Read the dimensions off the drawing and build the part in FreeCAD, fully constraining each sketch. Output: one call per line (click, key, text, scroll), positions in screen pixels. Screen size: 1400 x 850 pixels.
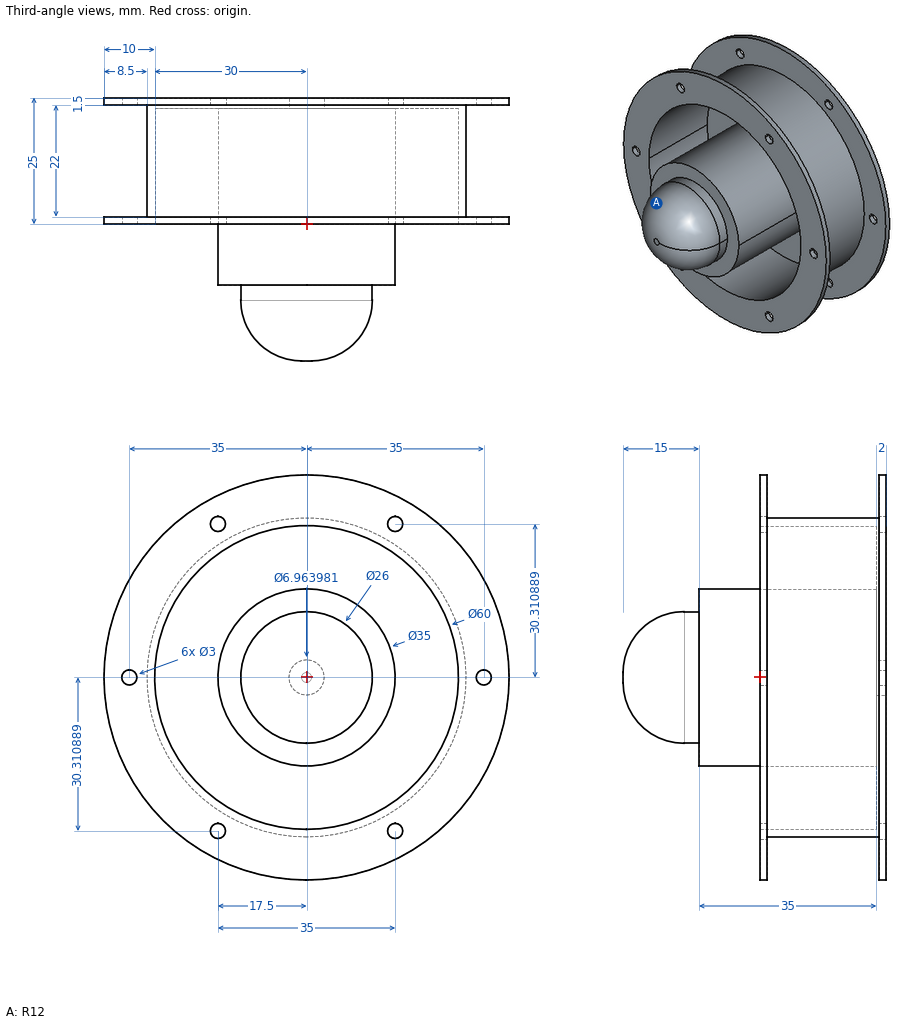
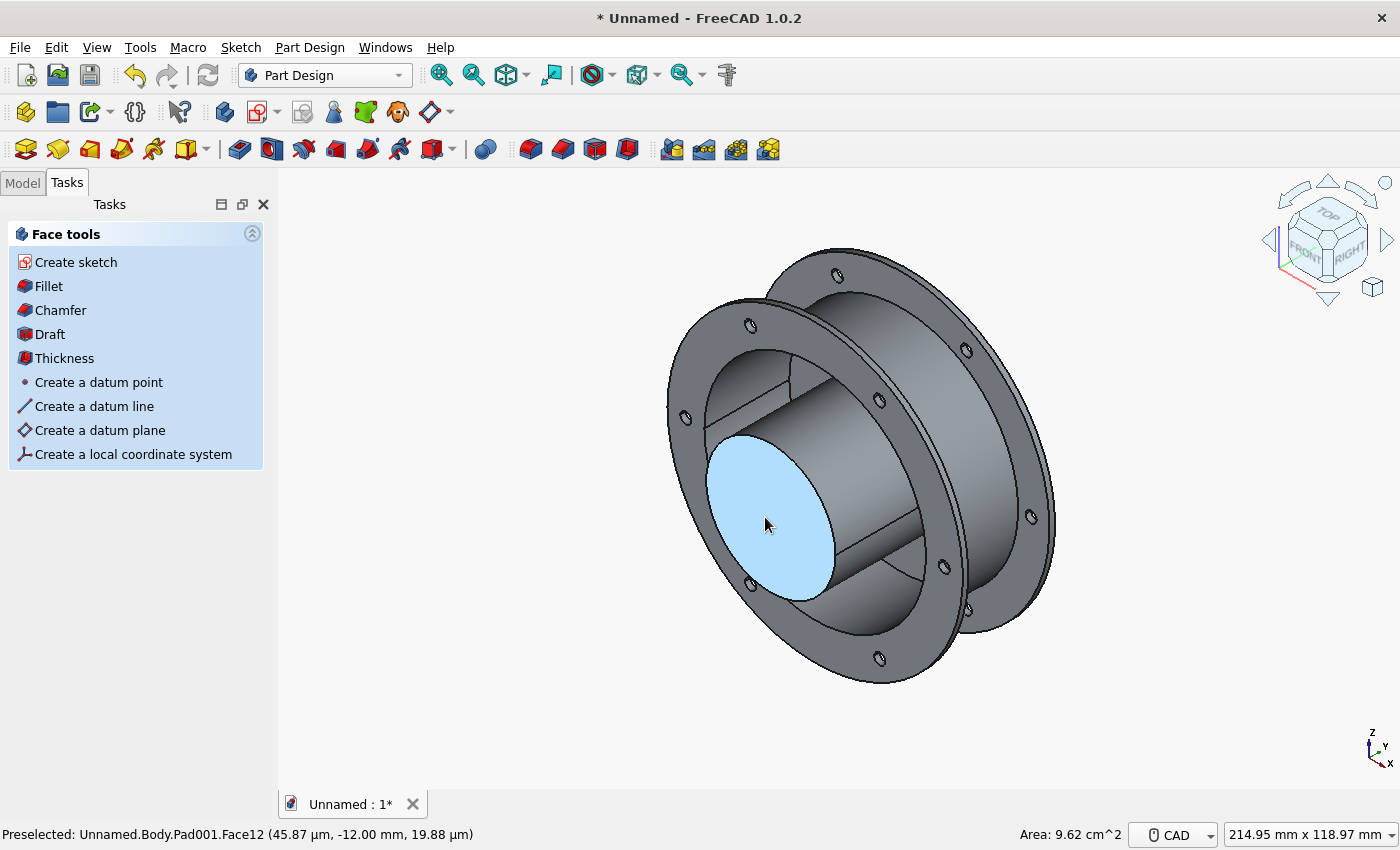
click(258, 112)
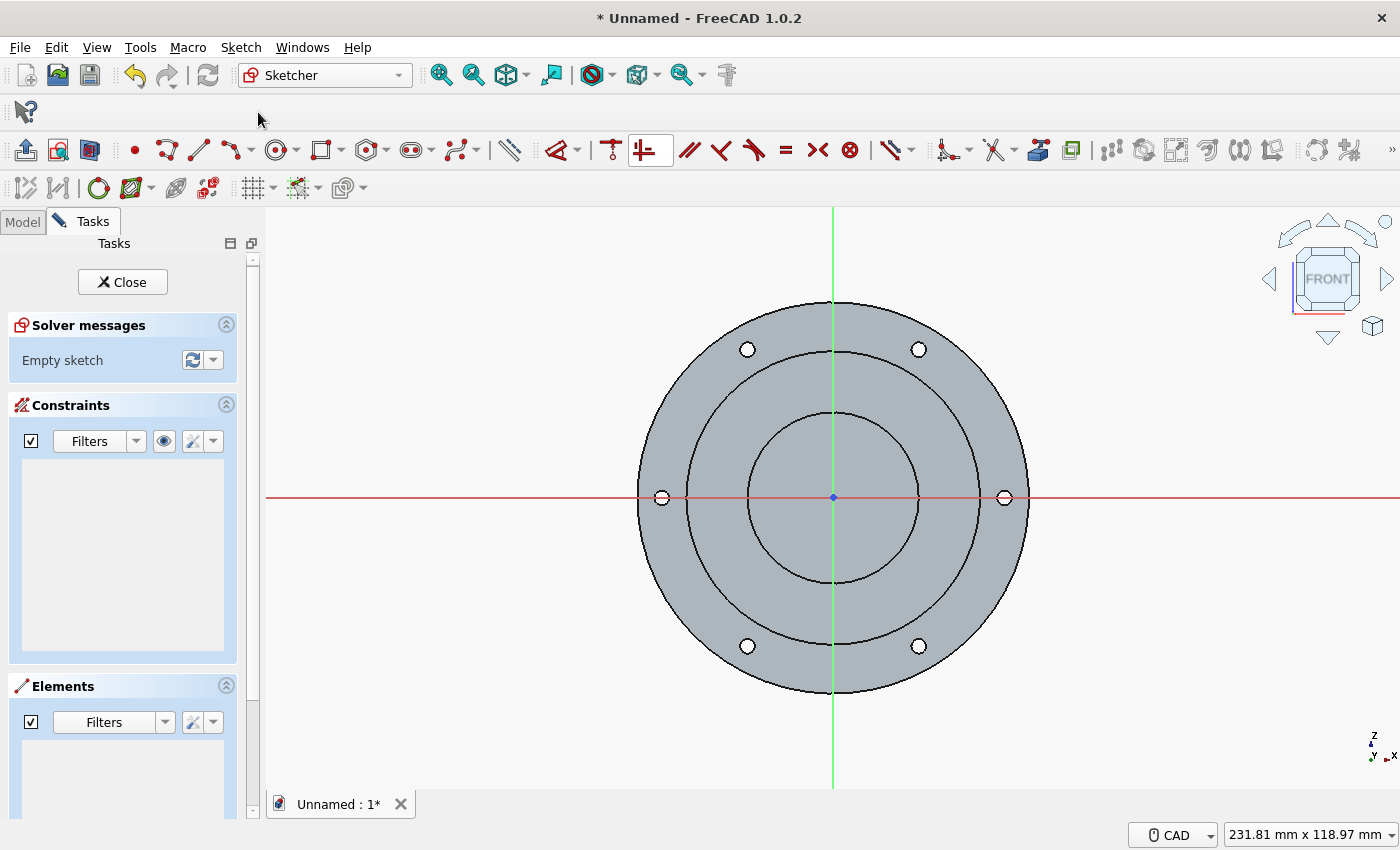
scroll(873, 498, up, 5)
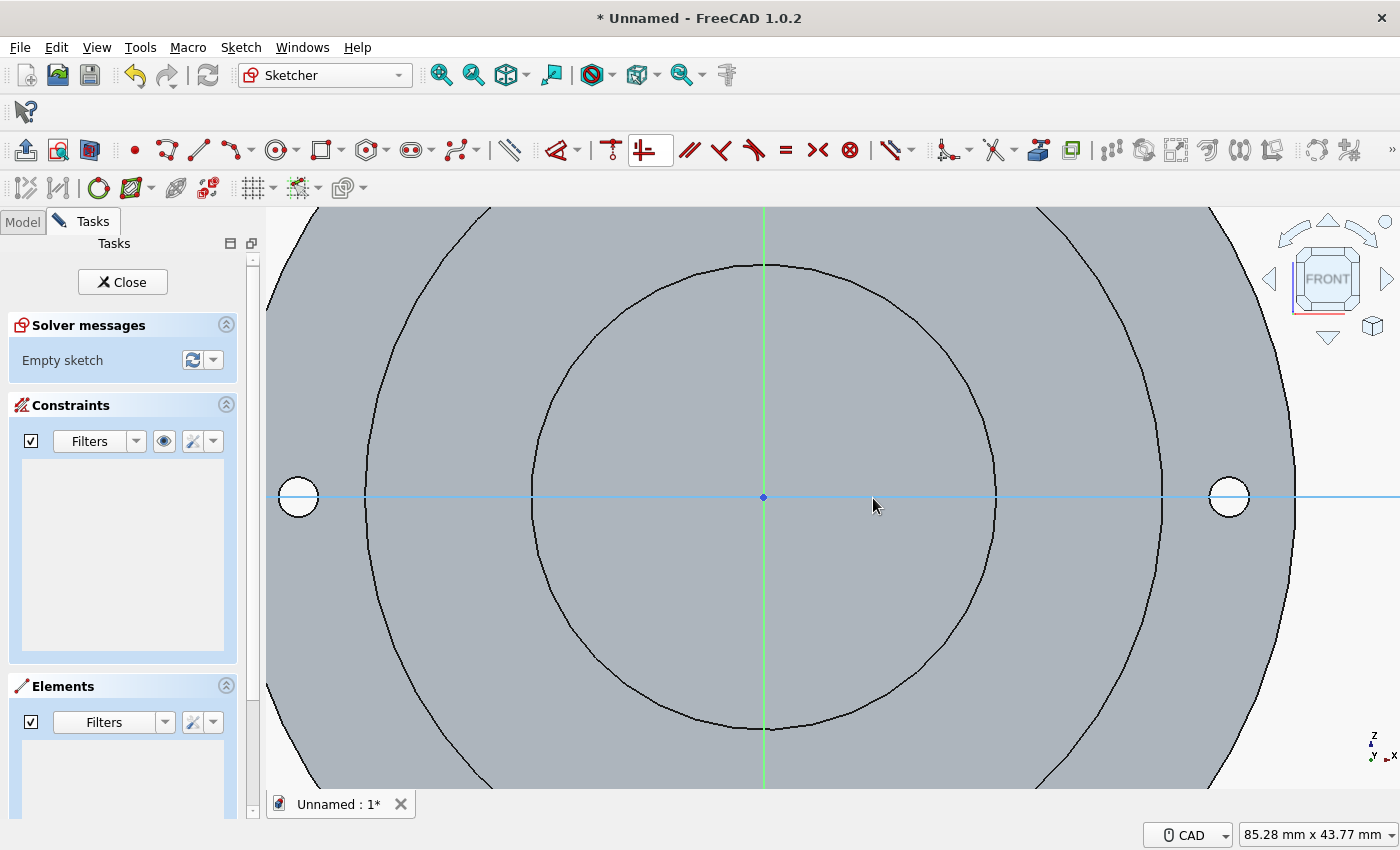
click(276, 150)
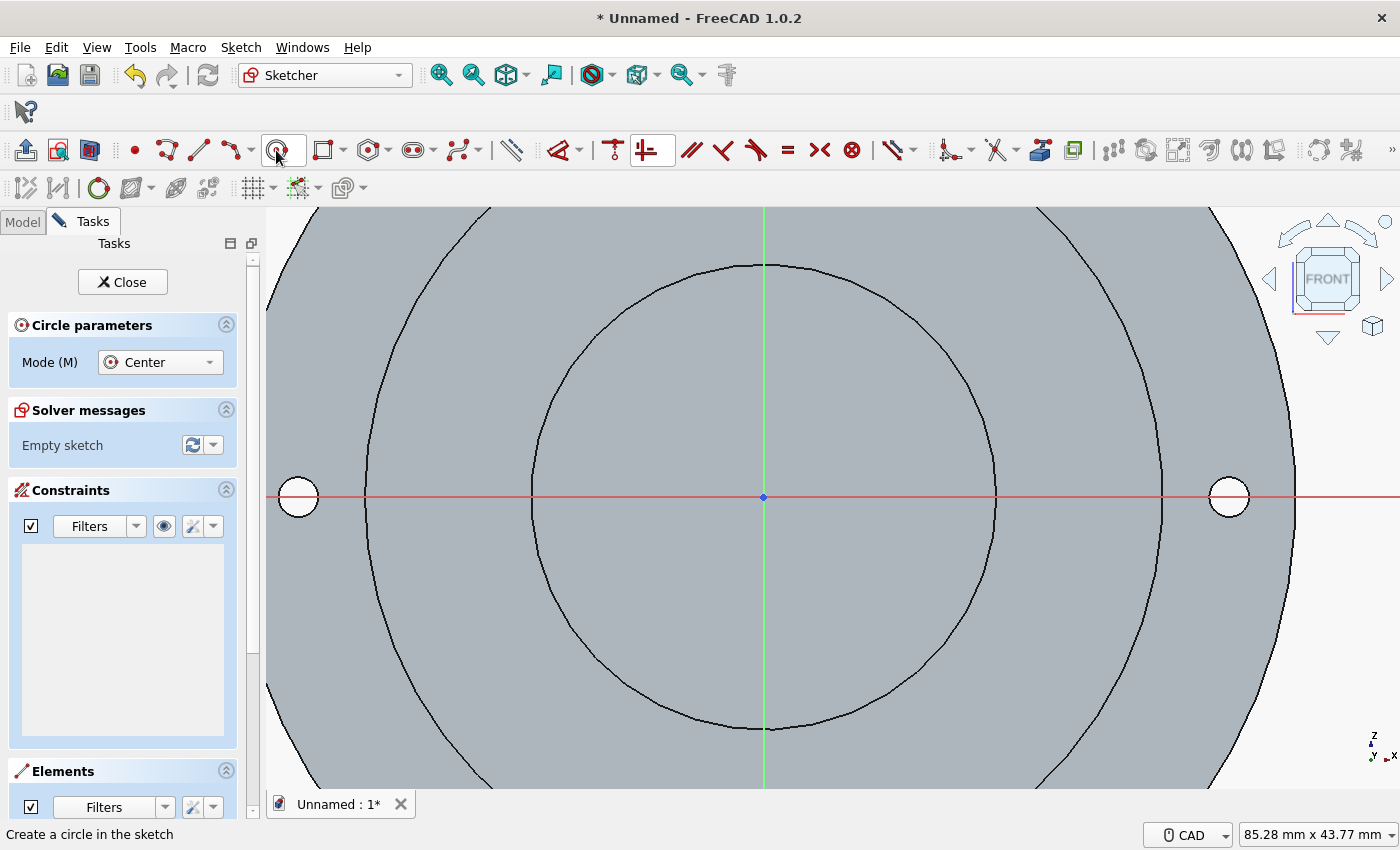
click(764, 497)
click(886, 375)
key(Escape)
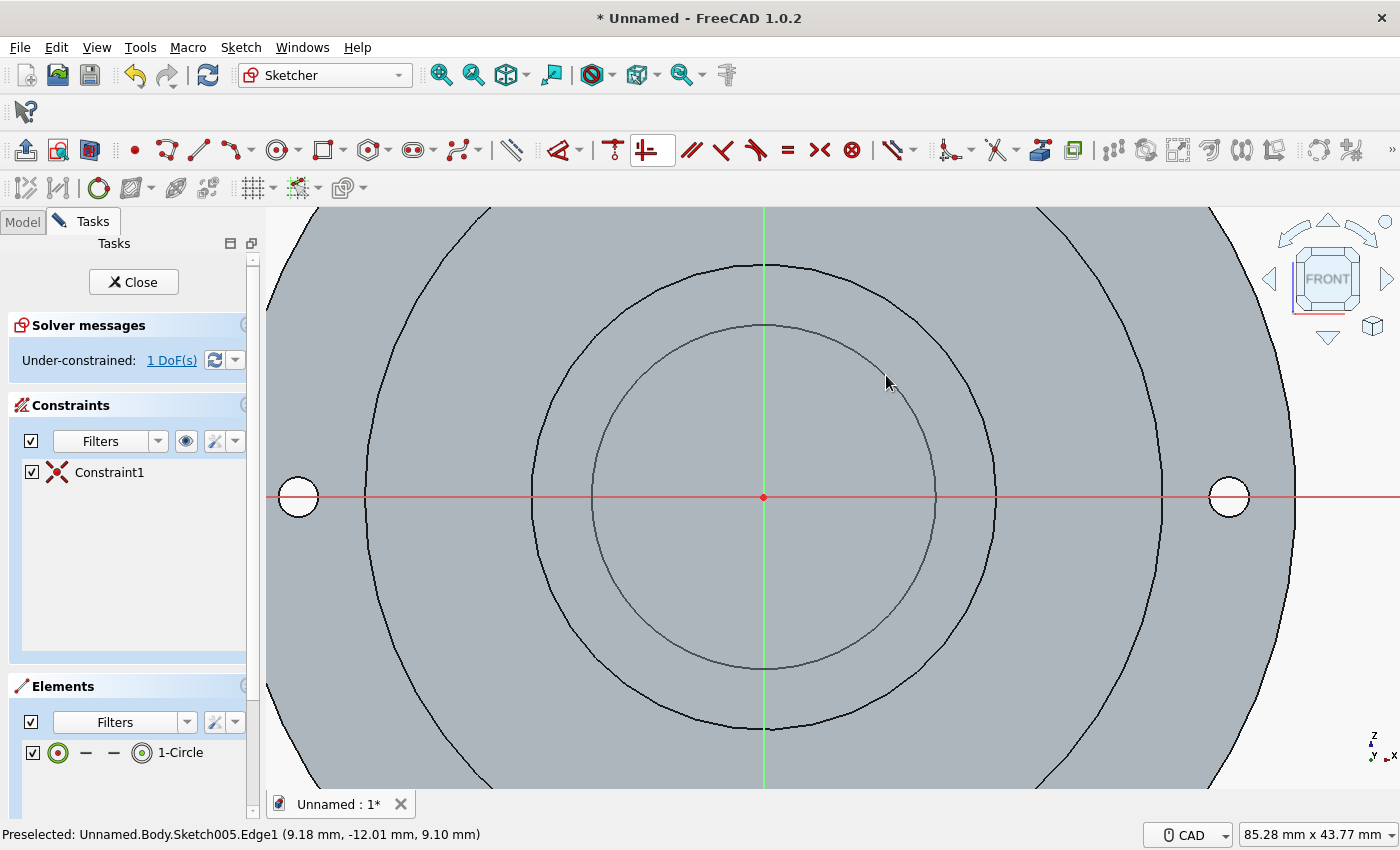
click(558, 150)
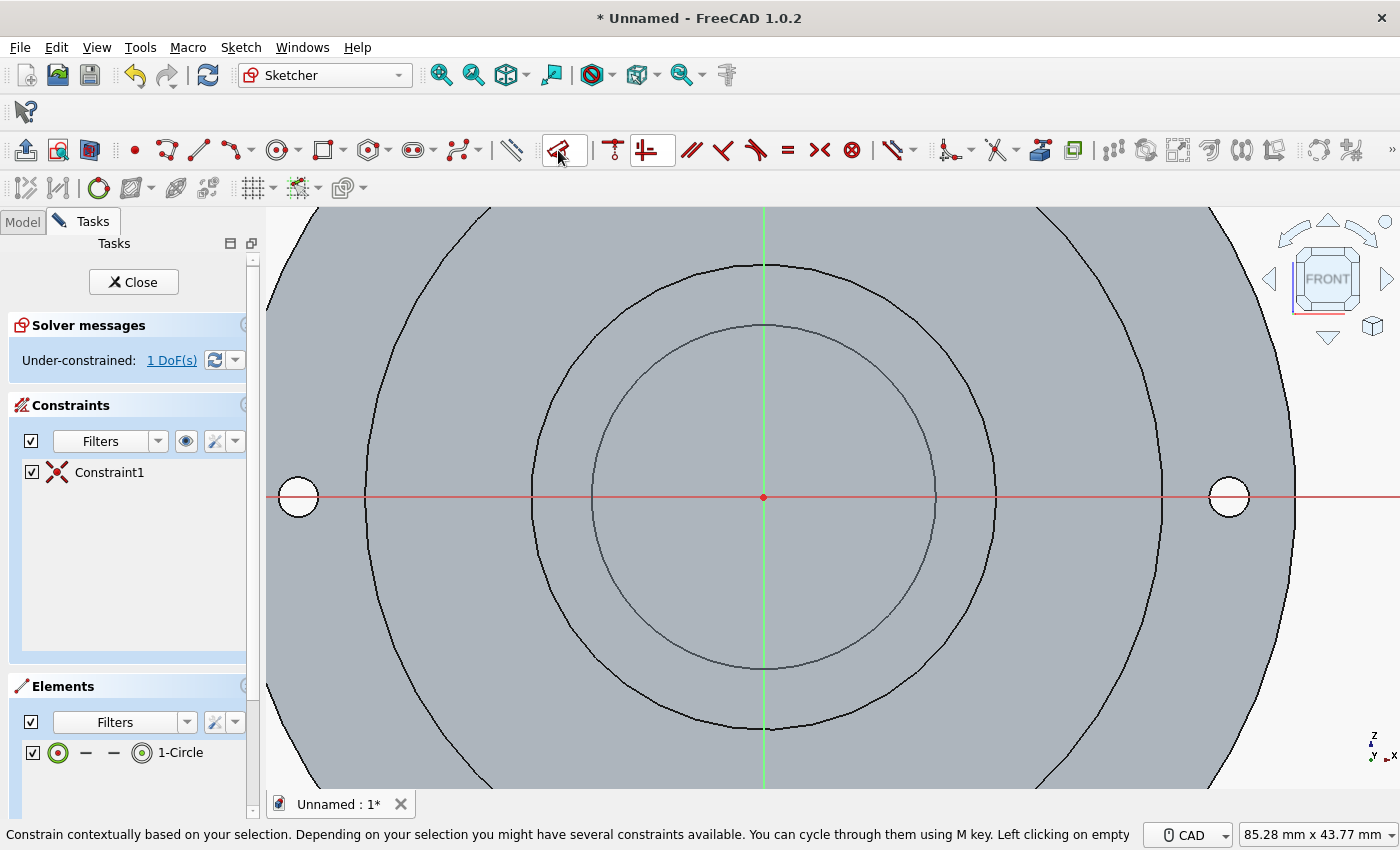
click(885, 375)
click(908, 352)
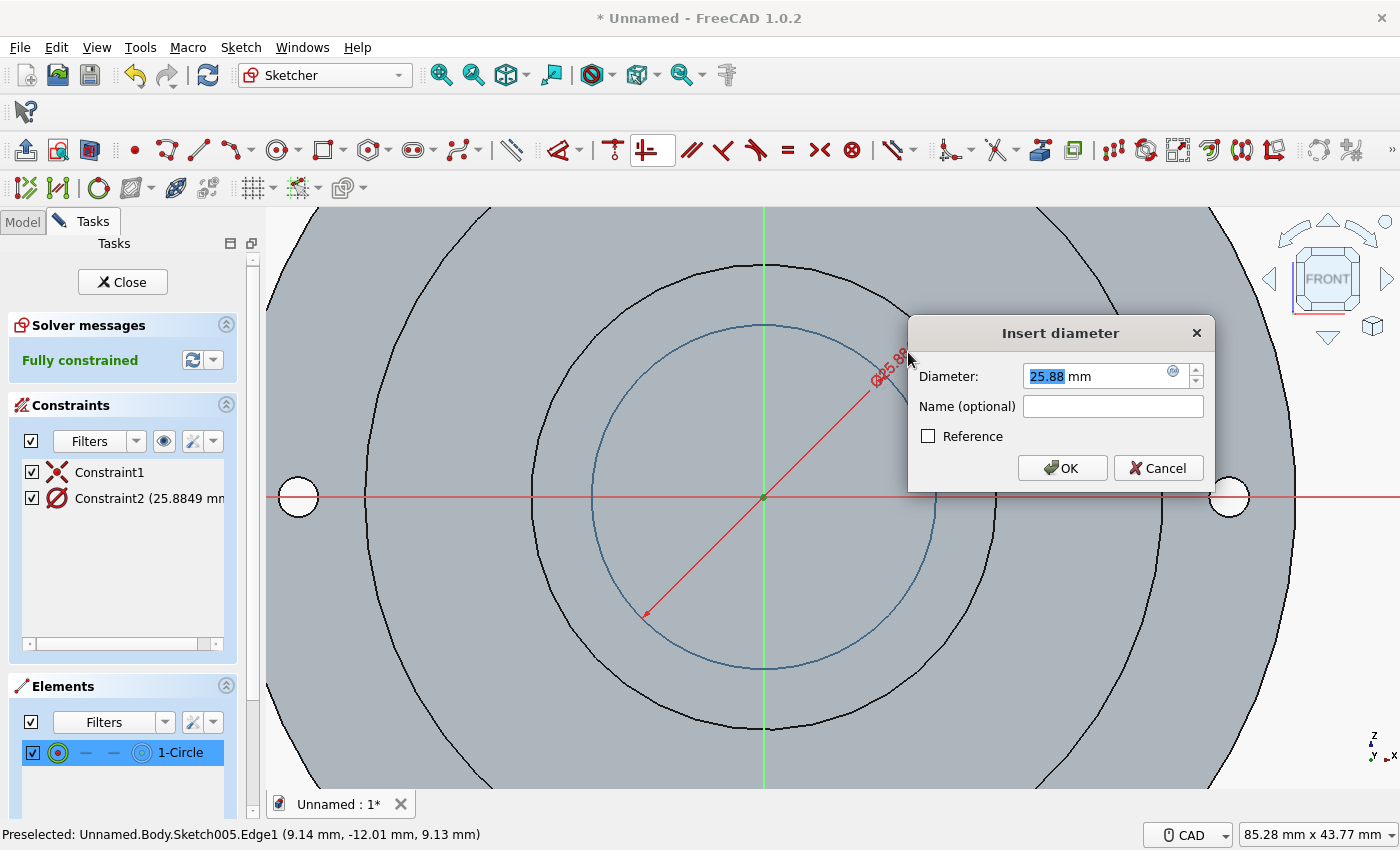
text(26)
key(Return)
key(Escape)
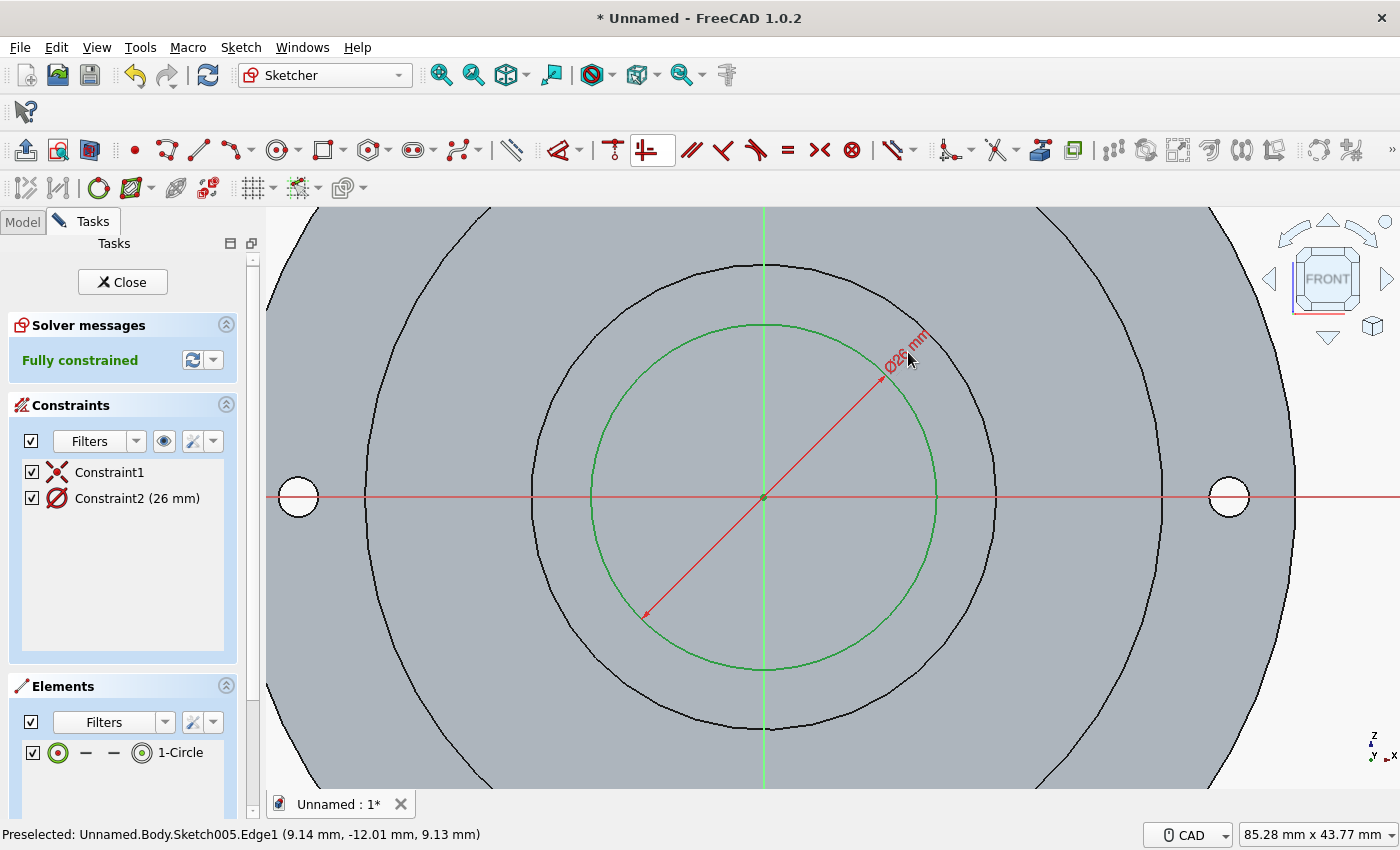
click(123, 282)